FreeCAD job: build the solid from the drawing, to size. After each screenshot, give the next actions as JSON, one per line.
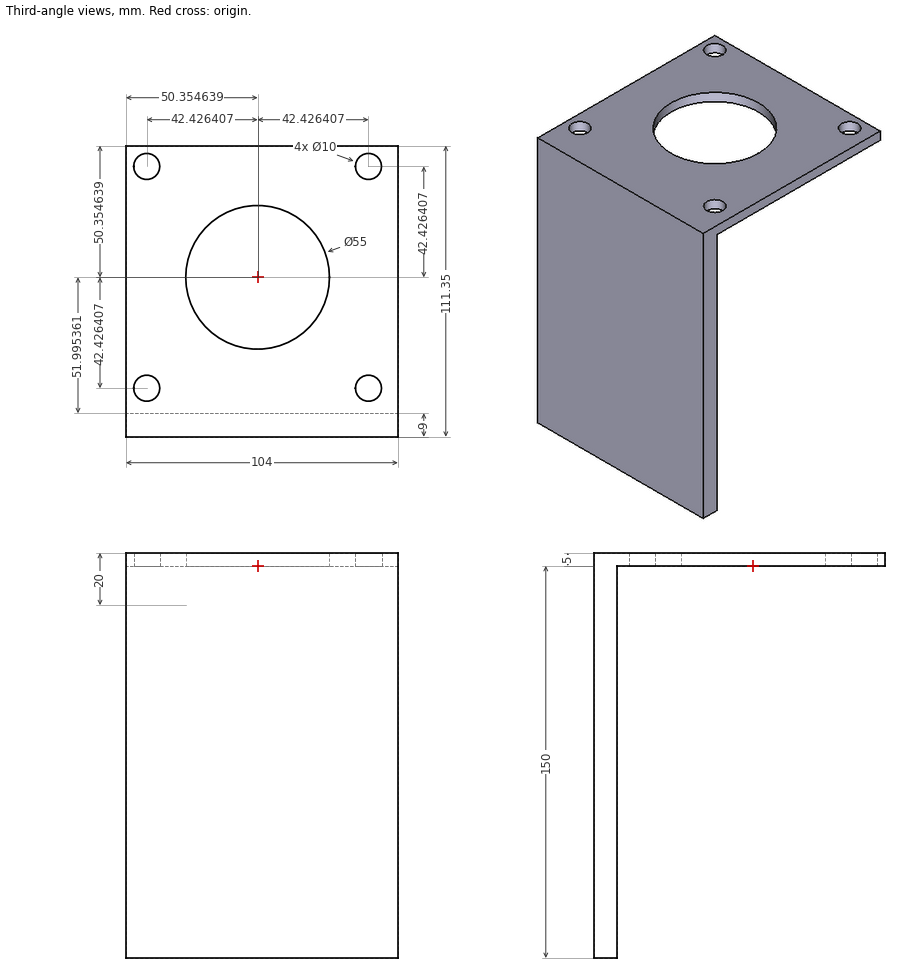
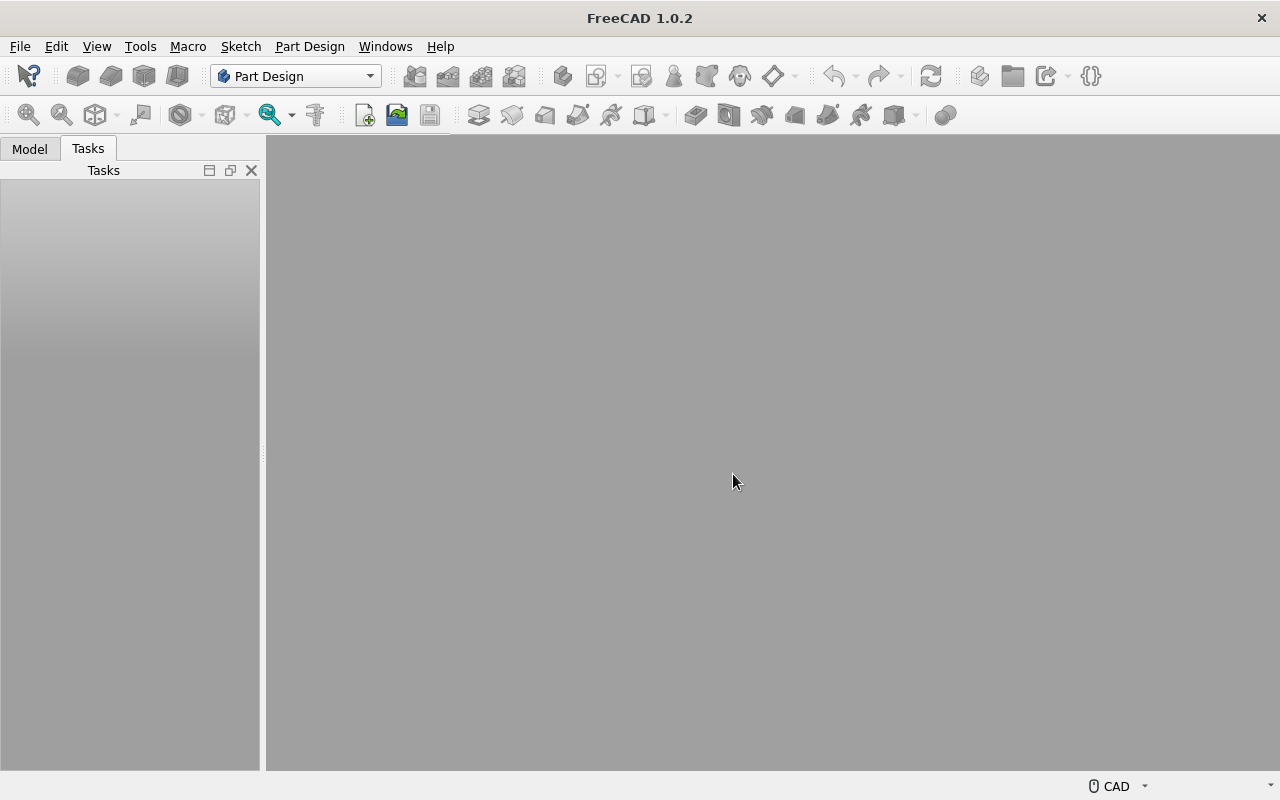
{"action": "left_click", "coordinate": [364, 116]}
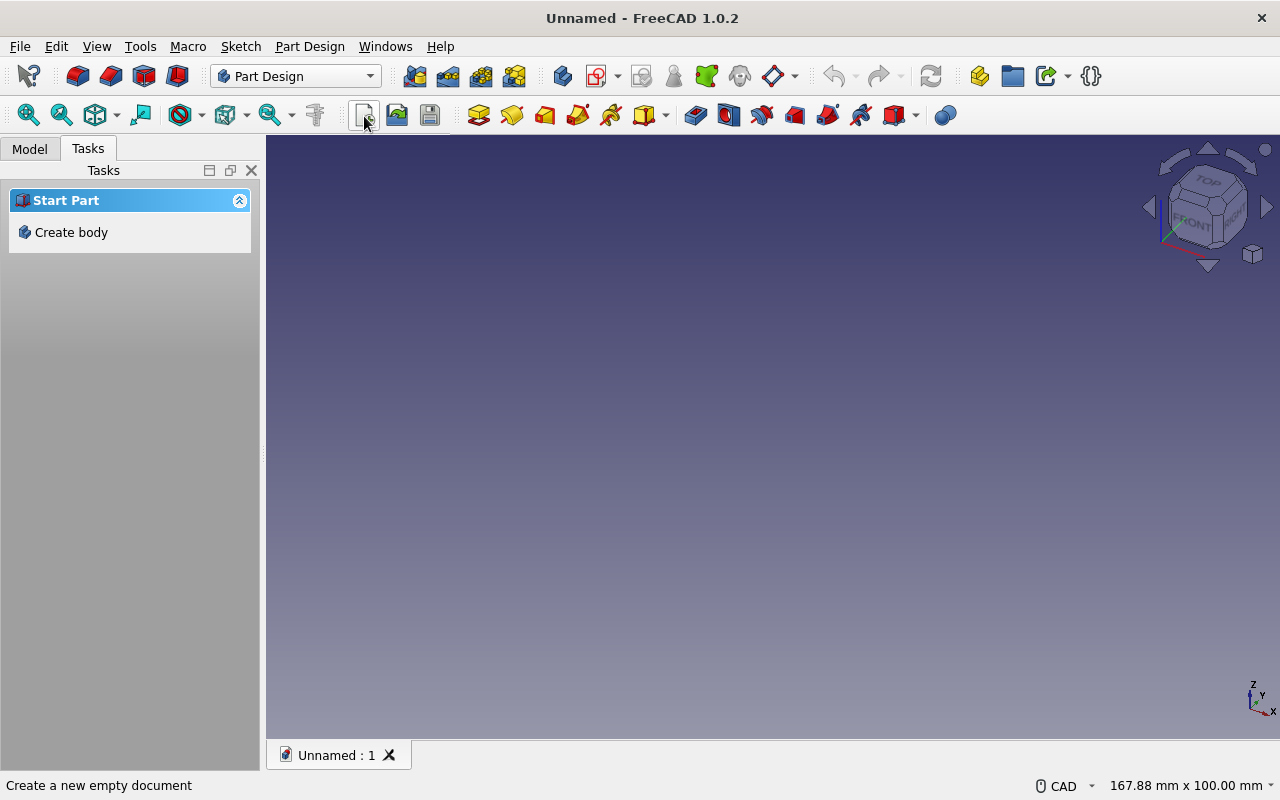
{"action": "left_click", "coordinate": [596, 76]}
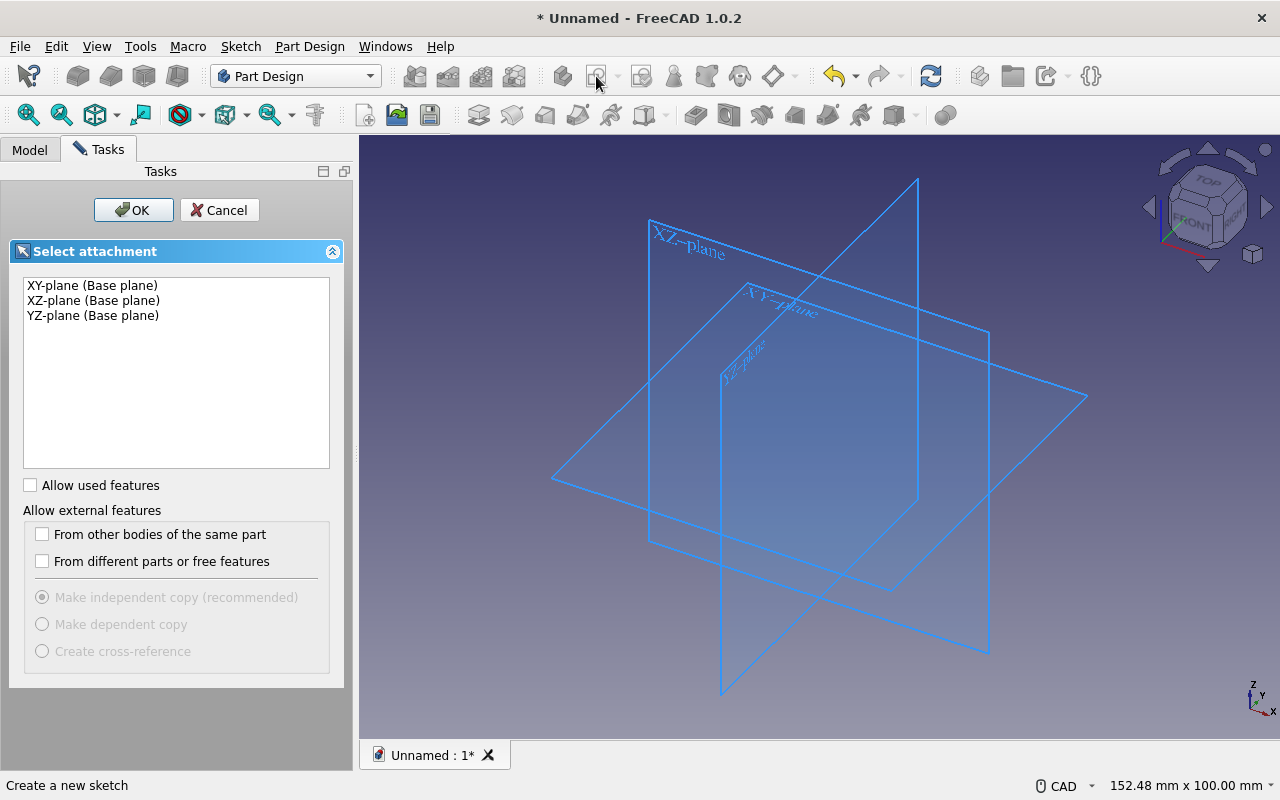
{"action": "left_click", "coordinate": [84, 286]}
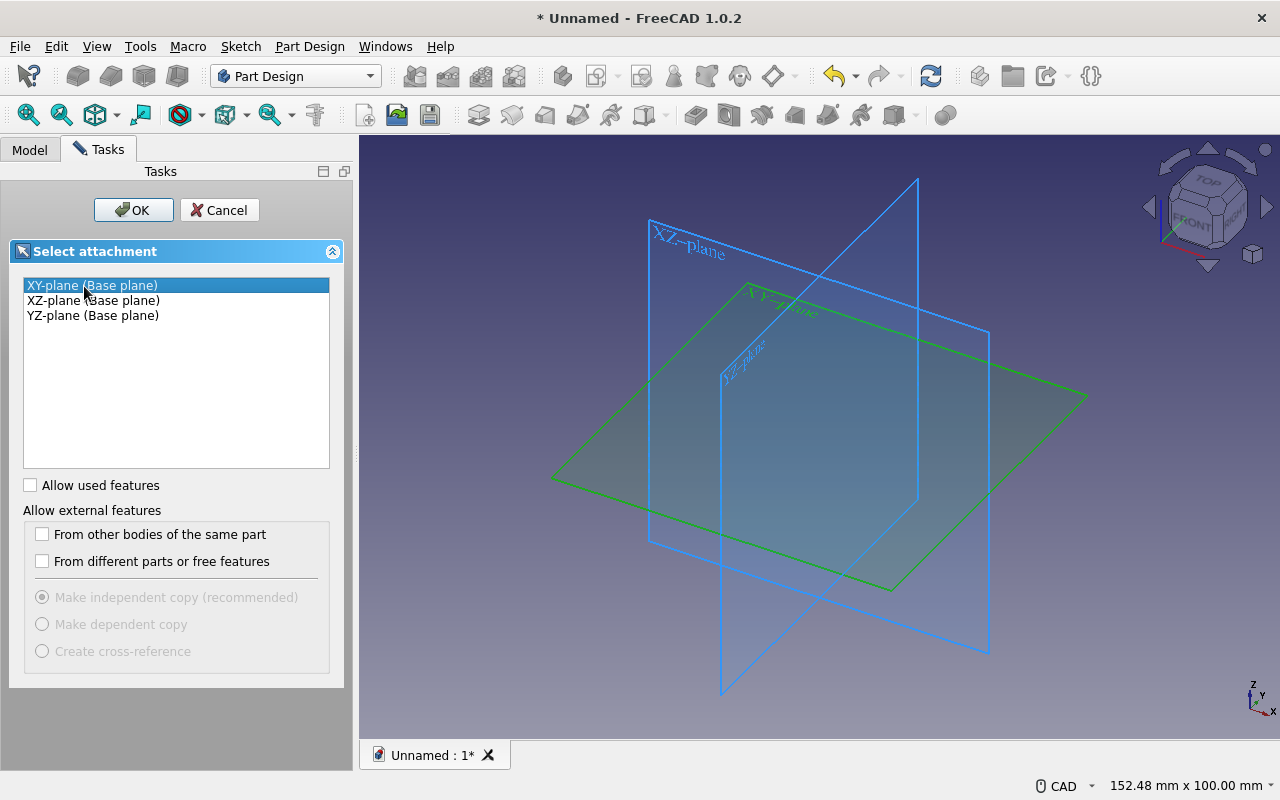
{"action": "left_click", "coordinate": [134, 210]}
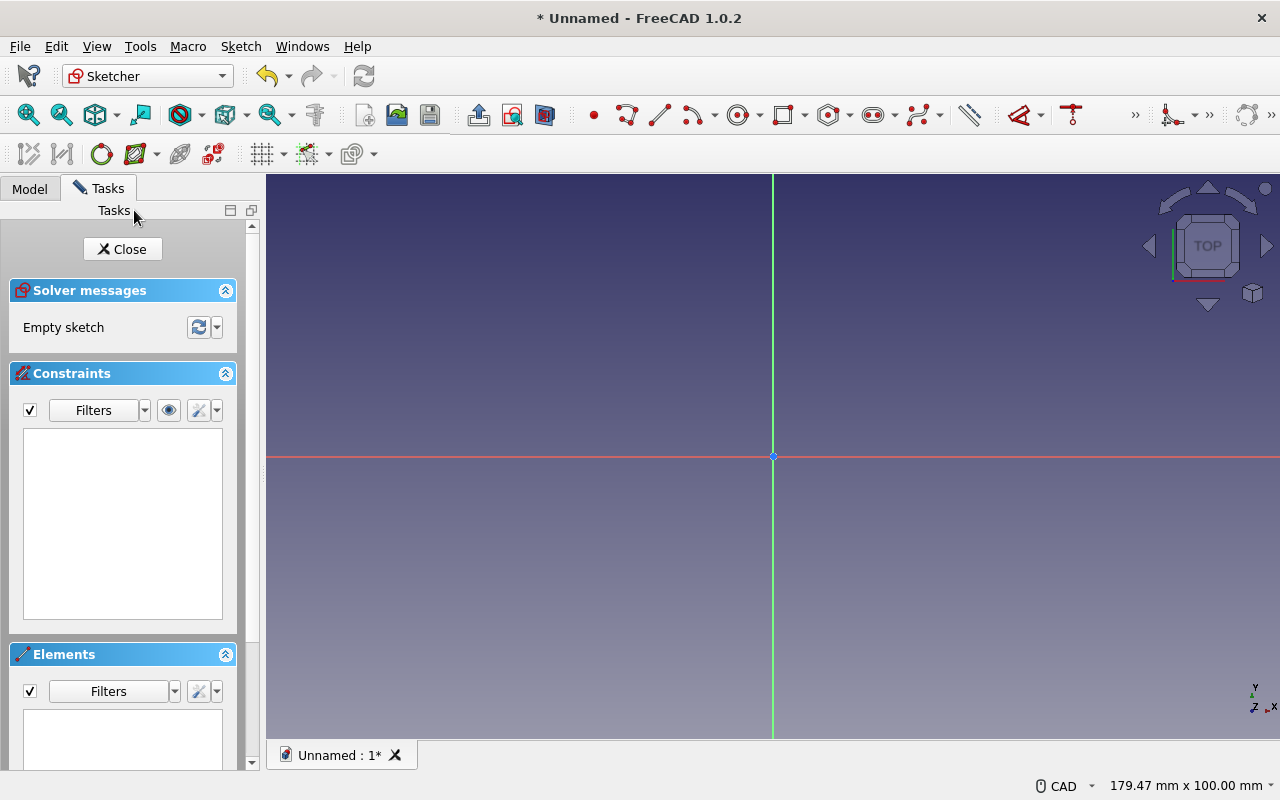
{"action": "scroll", "coordinate": [610, 420], "scroll_direction": "down", "scroll_amount": 3}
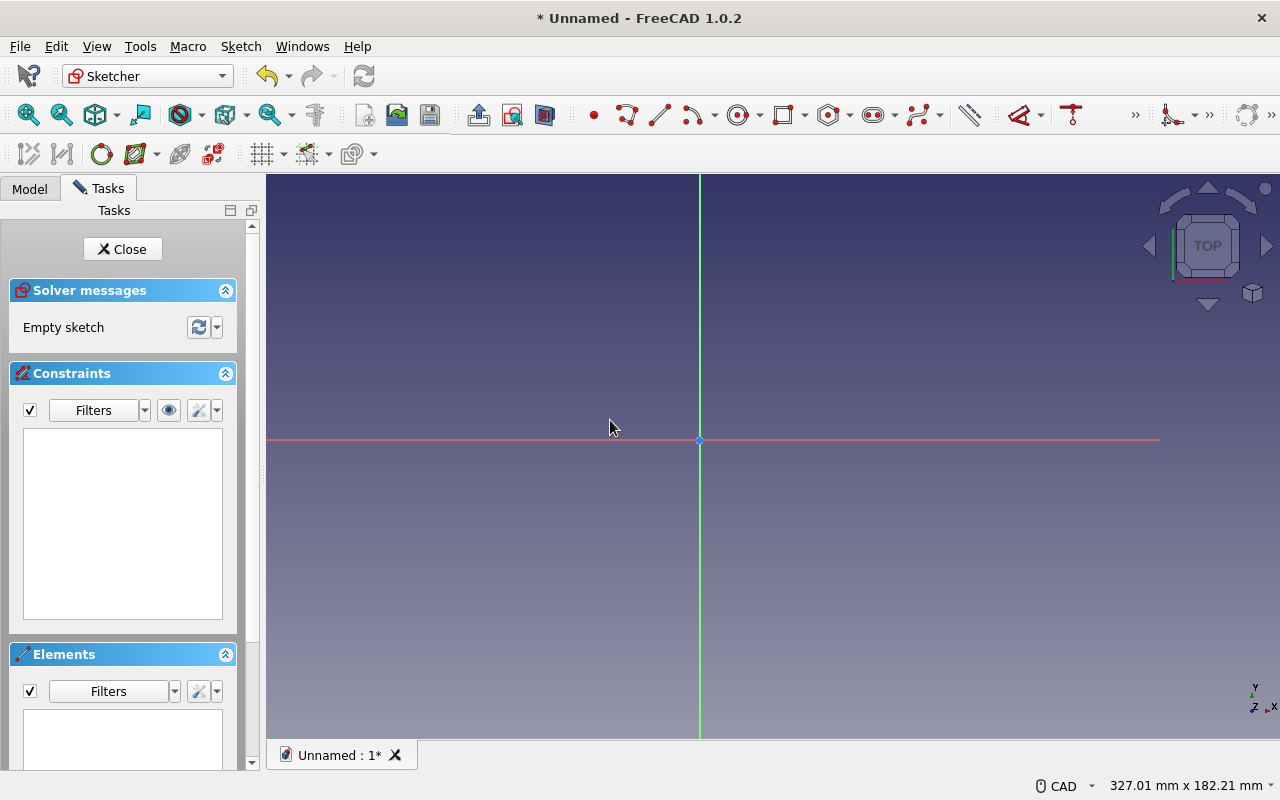
{"action": "left_click", "coordinate": [782, 116]}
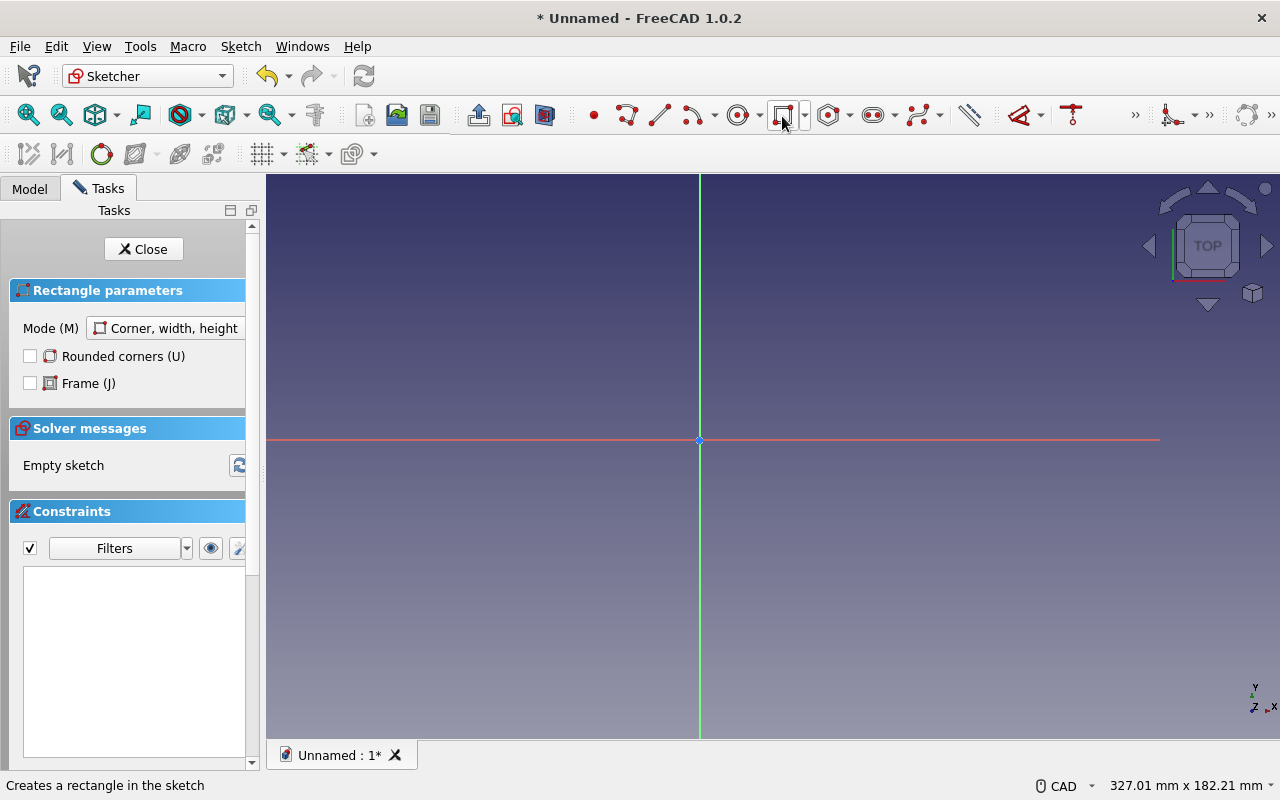
{"action": "left_click", "coordinate": [543, 284]}
{"action": "mouse_move", "coordinate": [866, 629]}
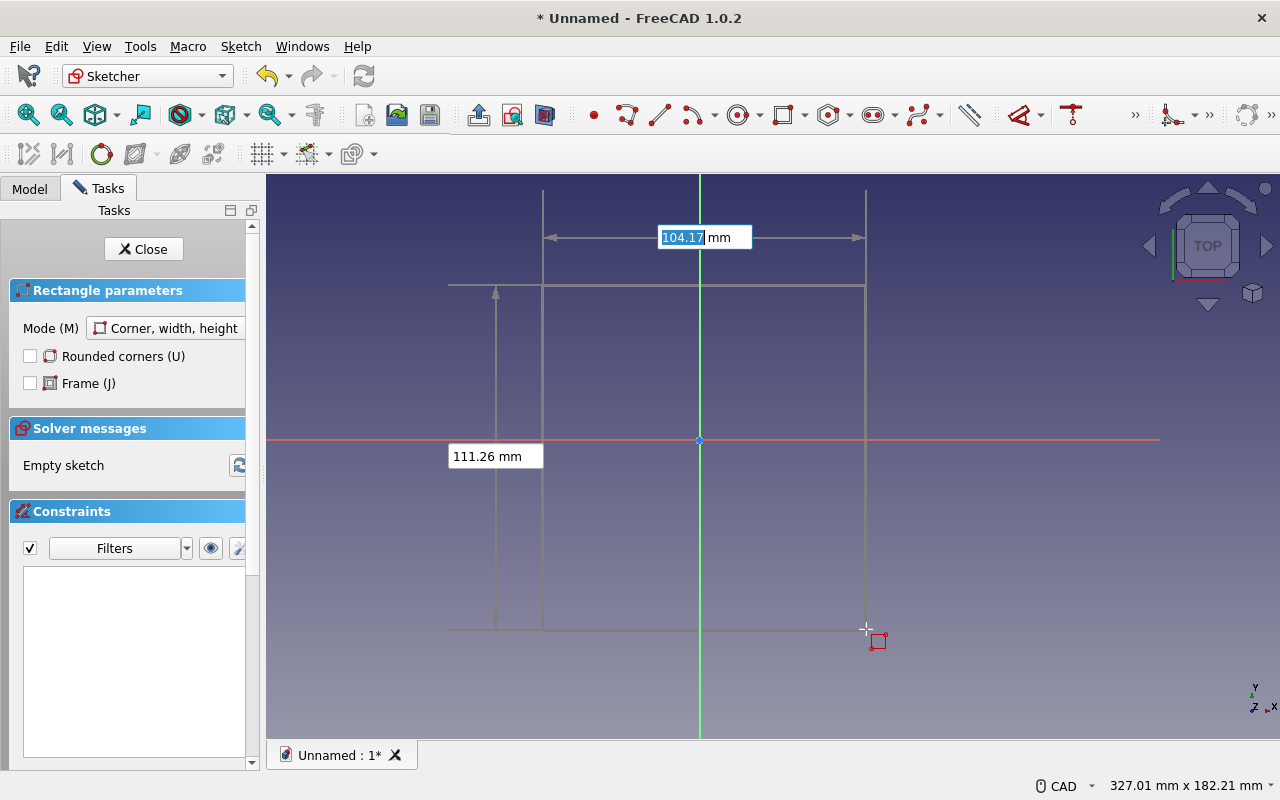
{"action": "type", "text": "104"}
{"action": "key", "text": "Tab"}
{"action": "type", "text": "111.35"}
{"action": "key", "text": "Return"}
{"action": "key", "text": "Escape"}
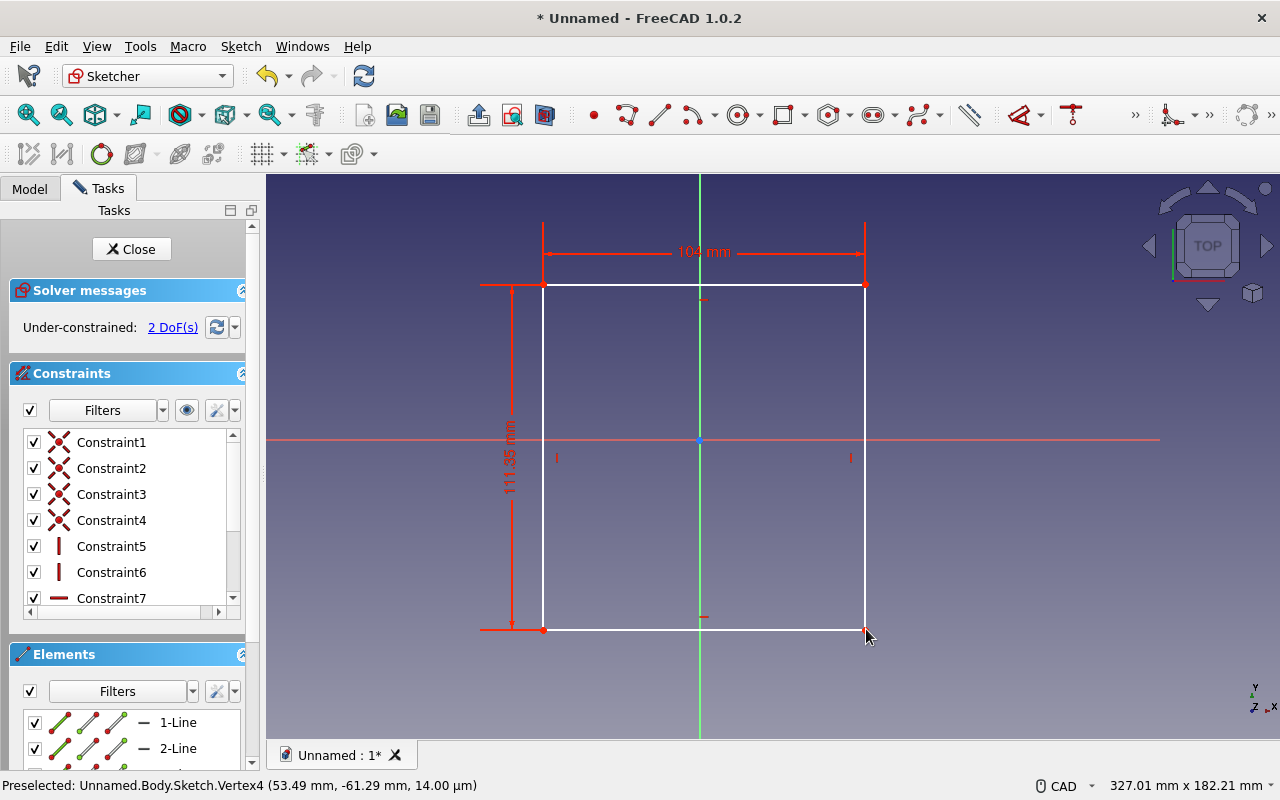
{"action": "left_click", "coordinate": [543, 285]}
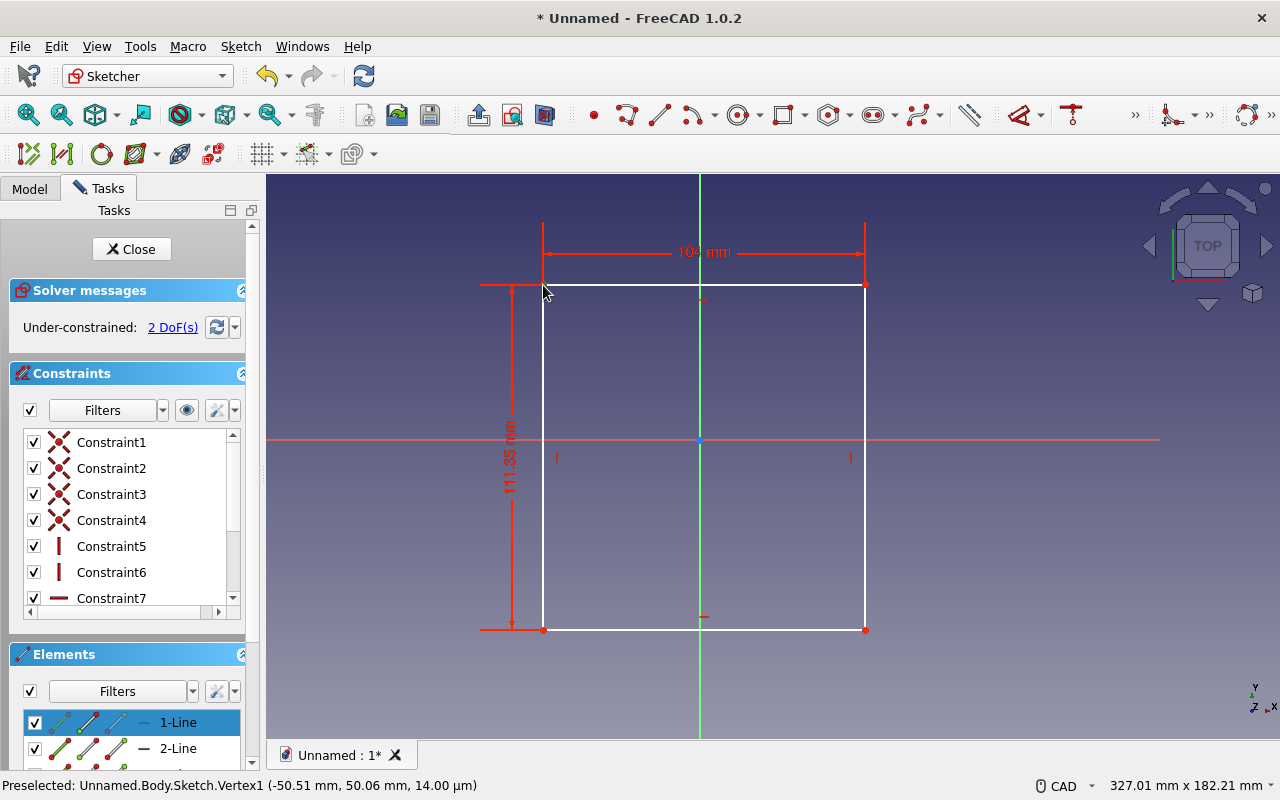
{"action": "left_click", "coordinate": [1040, 116]}